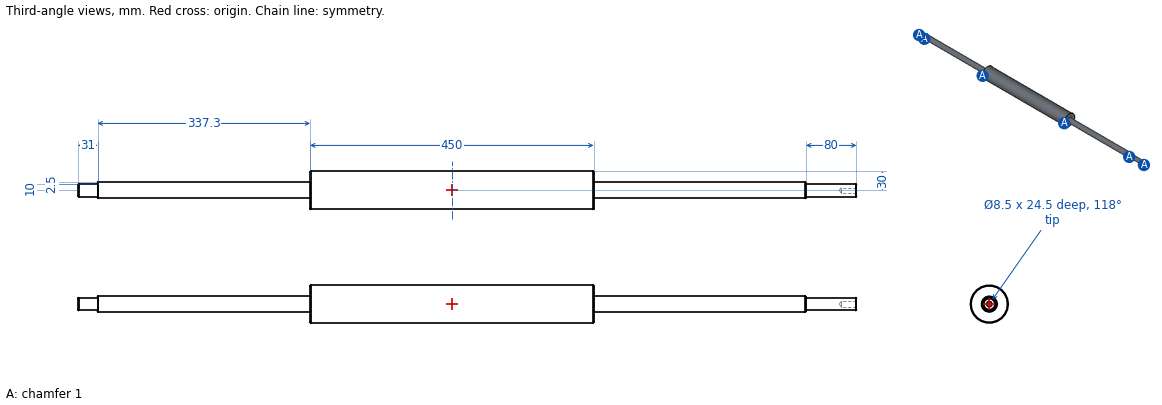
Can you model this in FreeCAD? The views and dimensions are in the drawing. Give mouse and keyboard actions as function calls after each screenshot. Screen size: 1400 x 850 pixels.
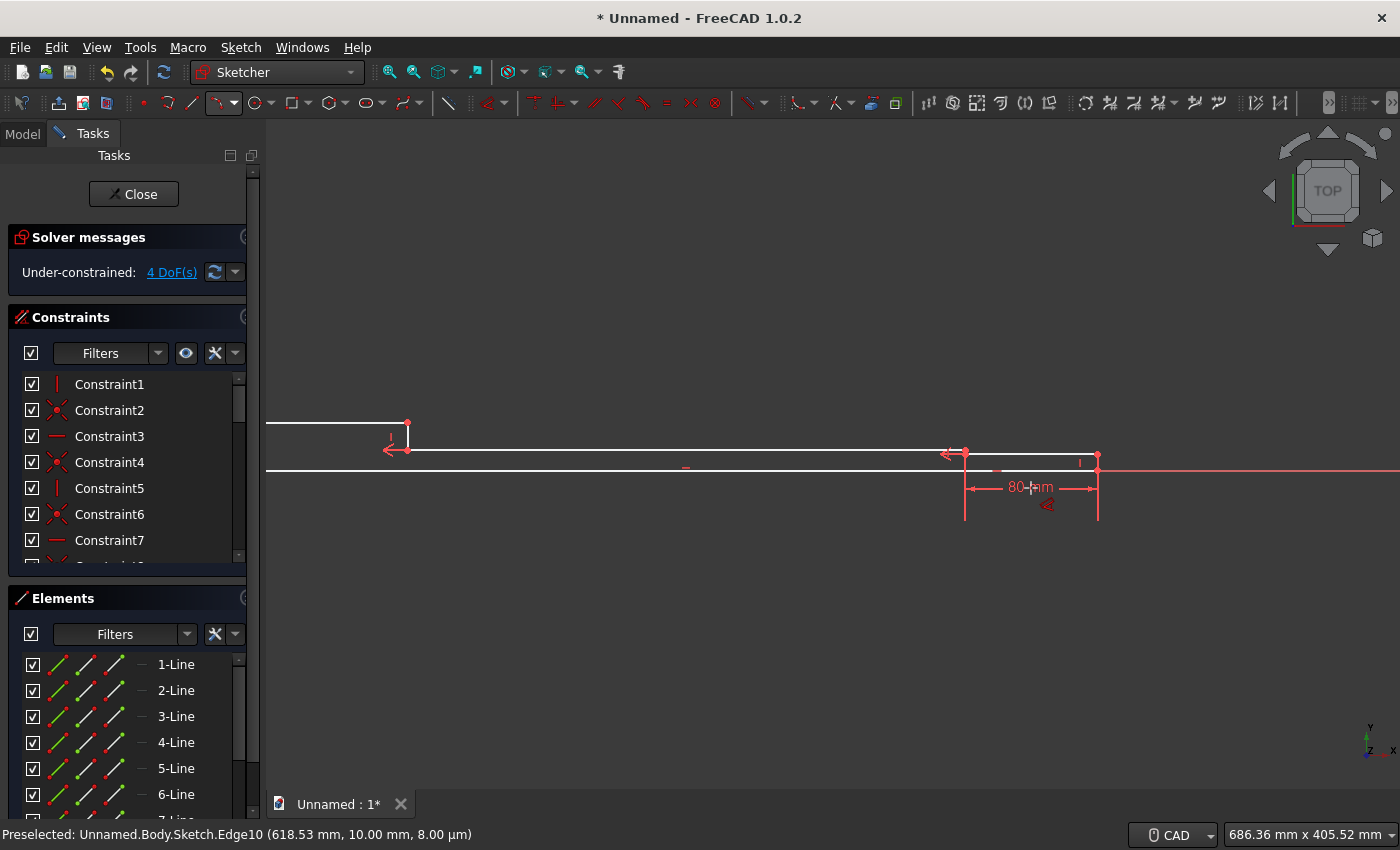
scroll(1061, 457, down, 6)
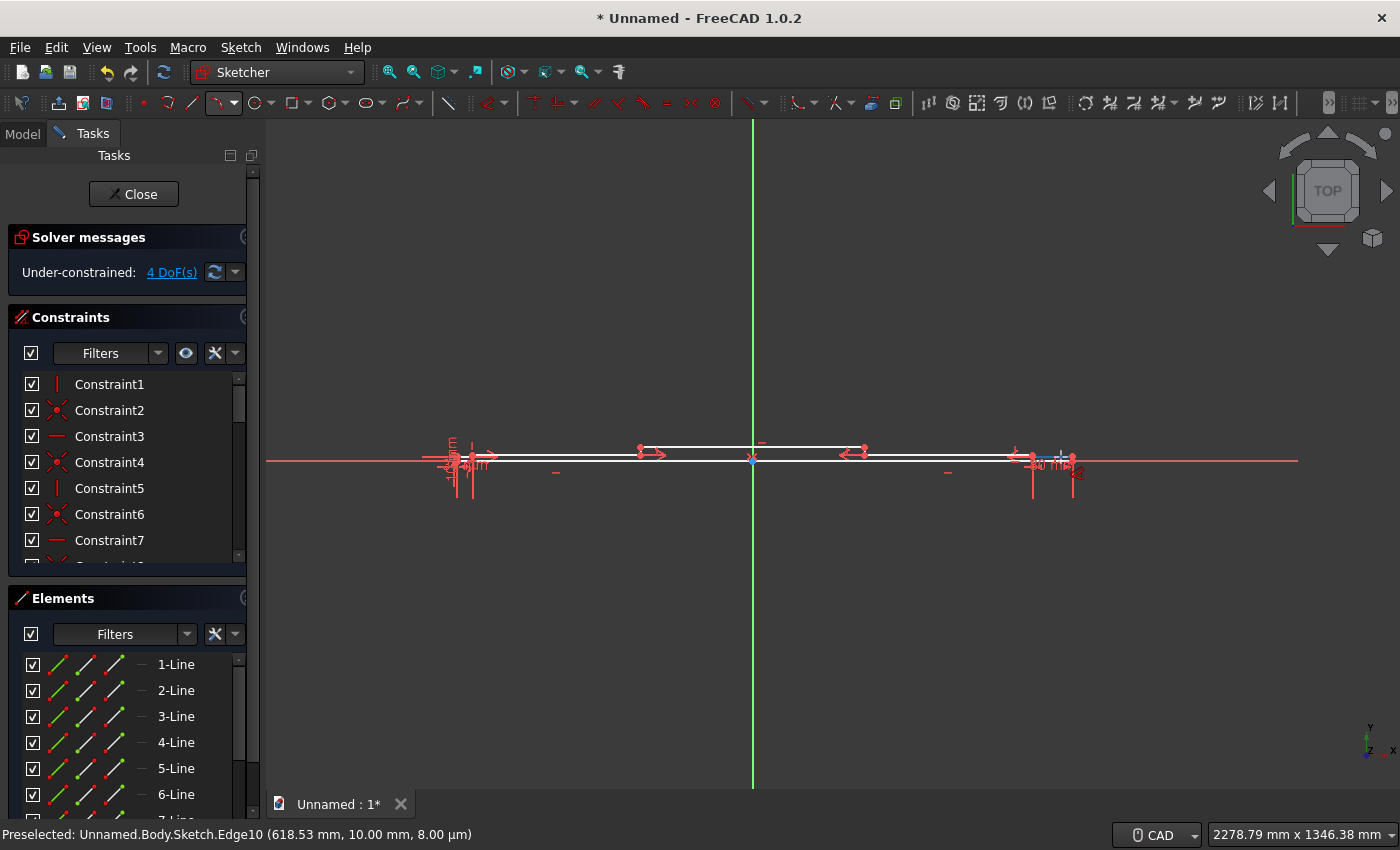
click(798, 447)
click(701, 413)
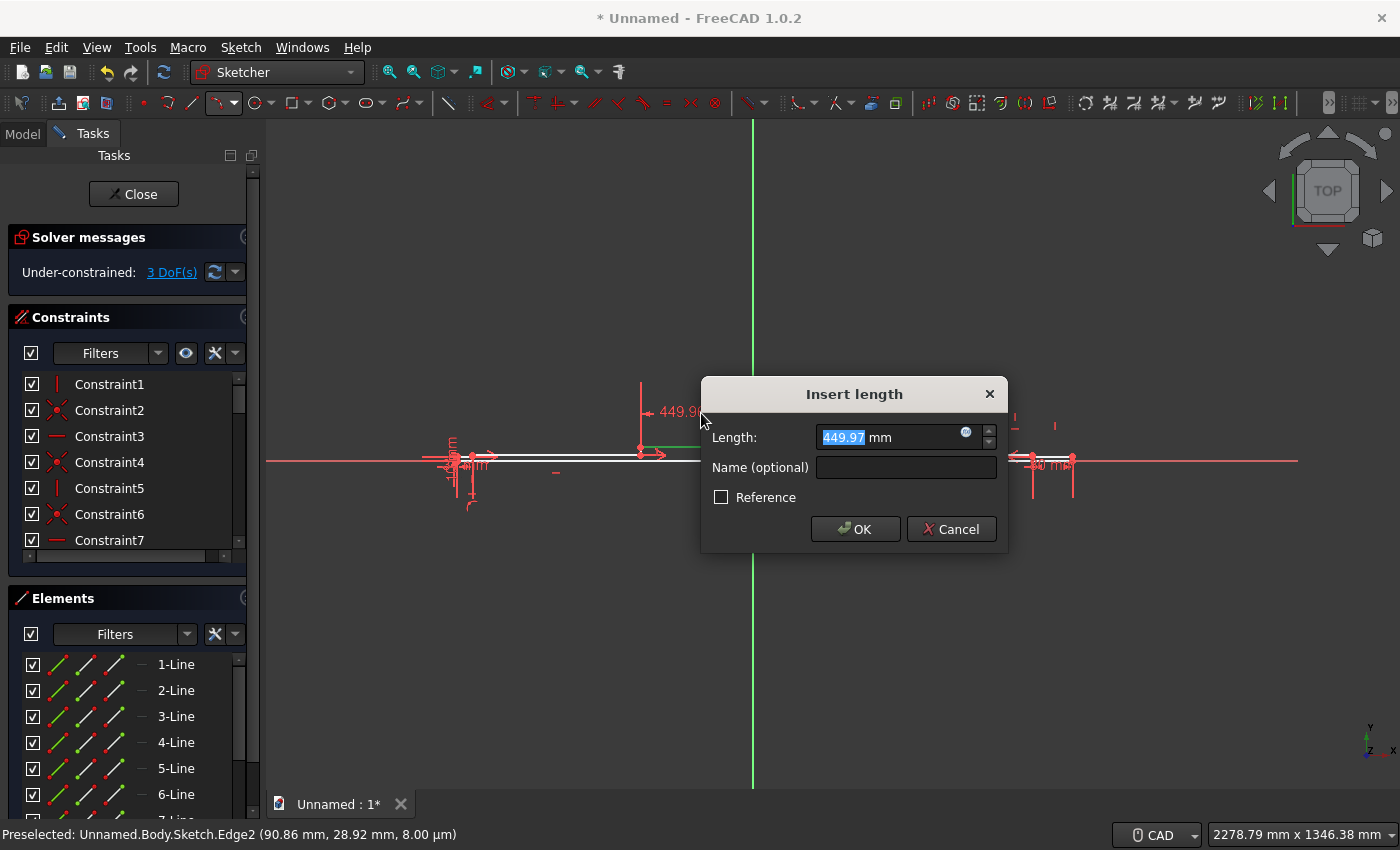
text(450)
key(Return)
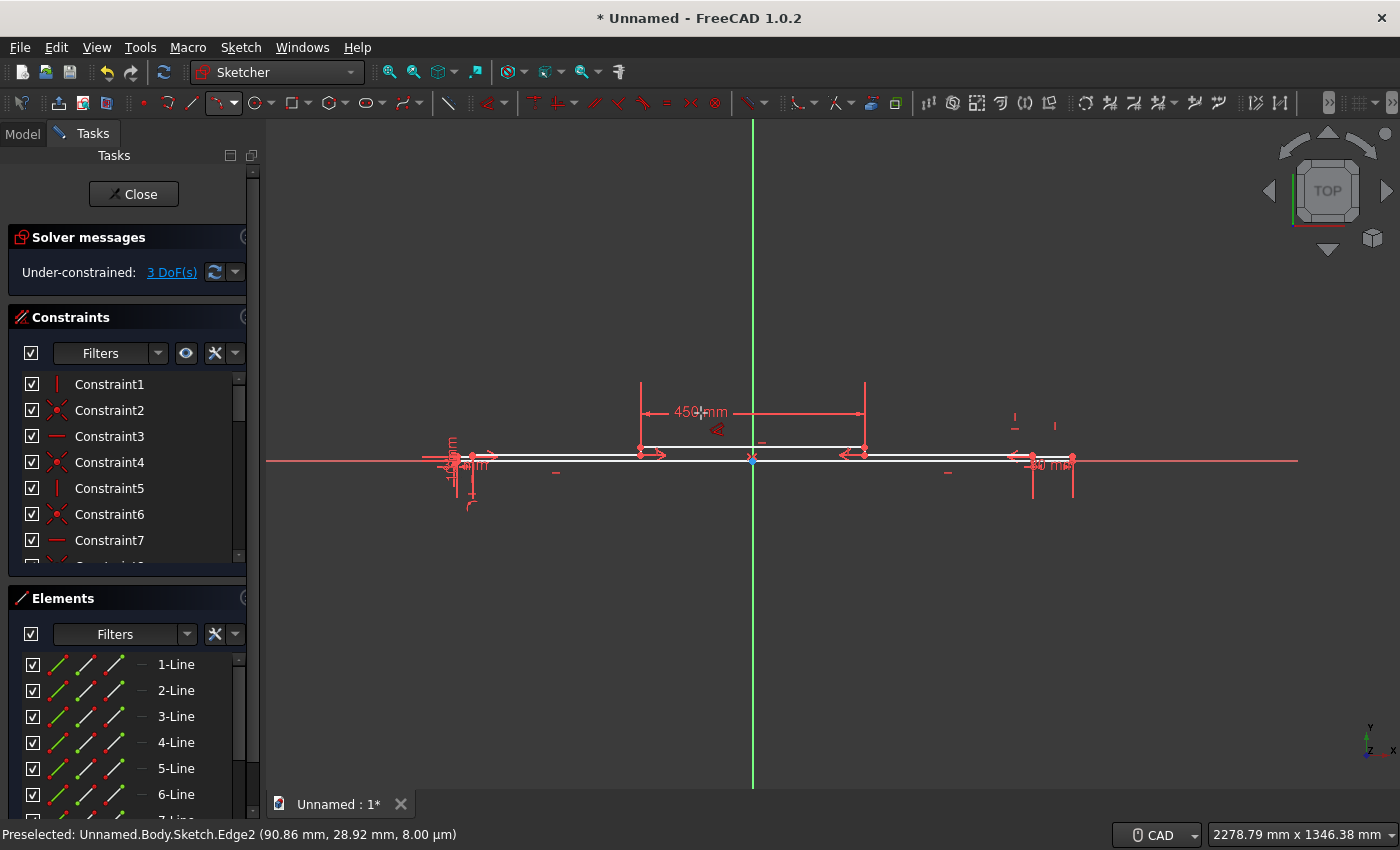
scroll(473, 456, up, 18)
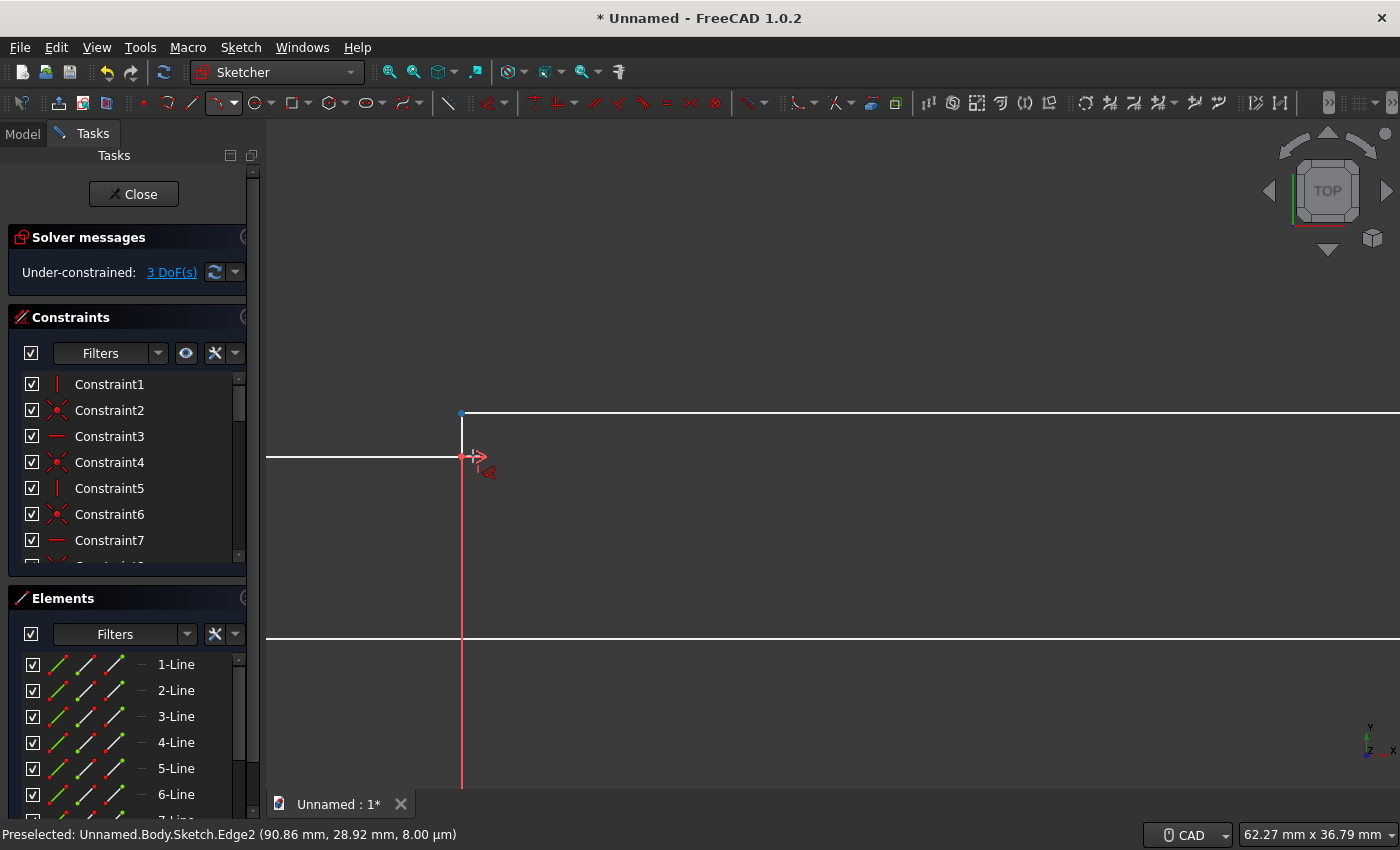
click(462, 435)
click(428, 435)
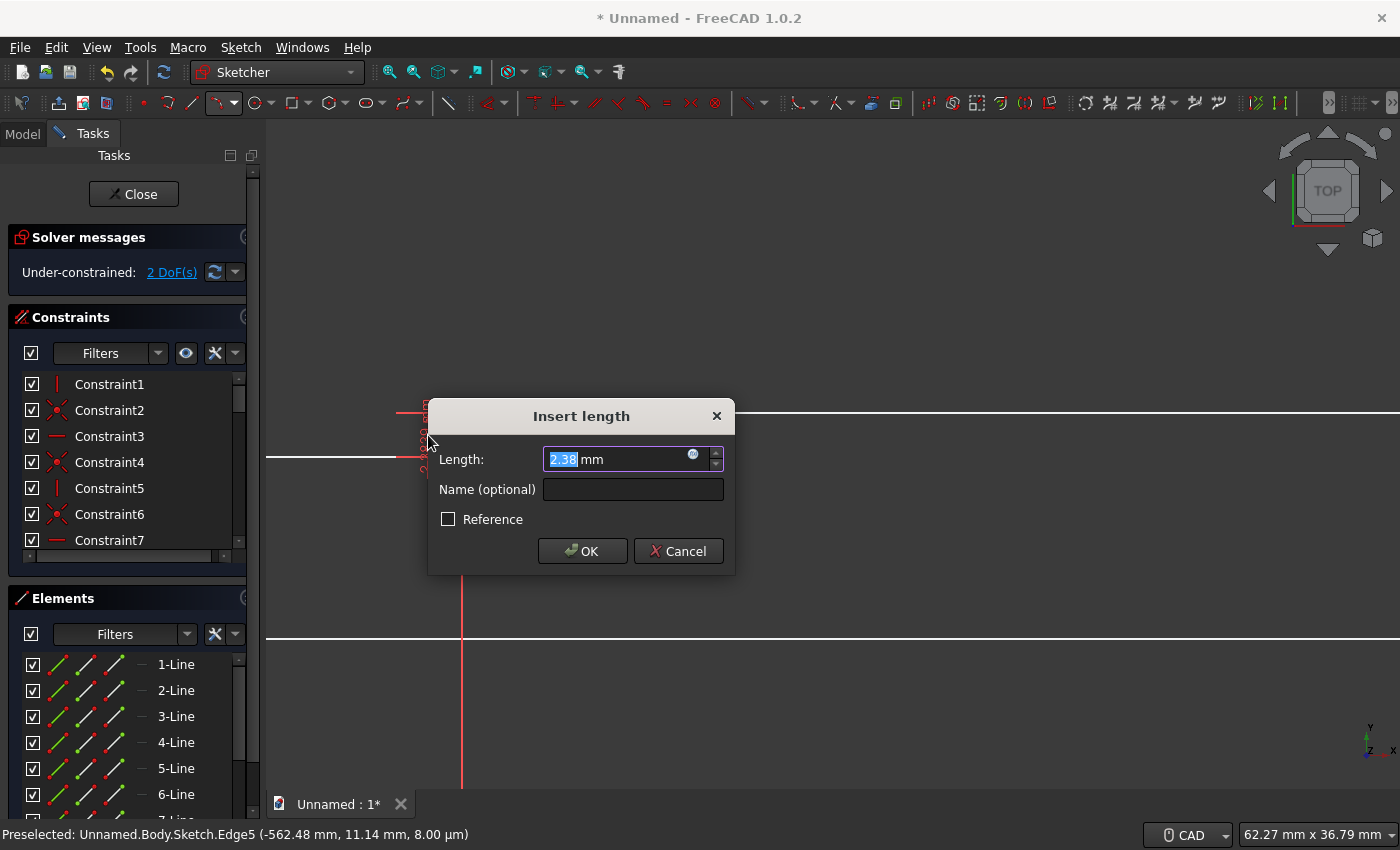
text(2.5)
key(Return)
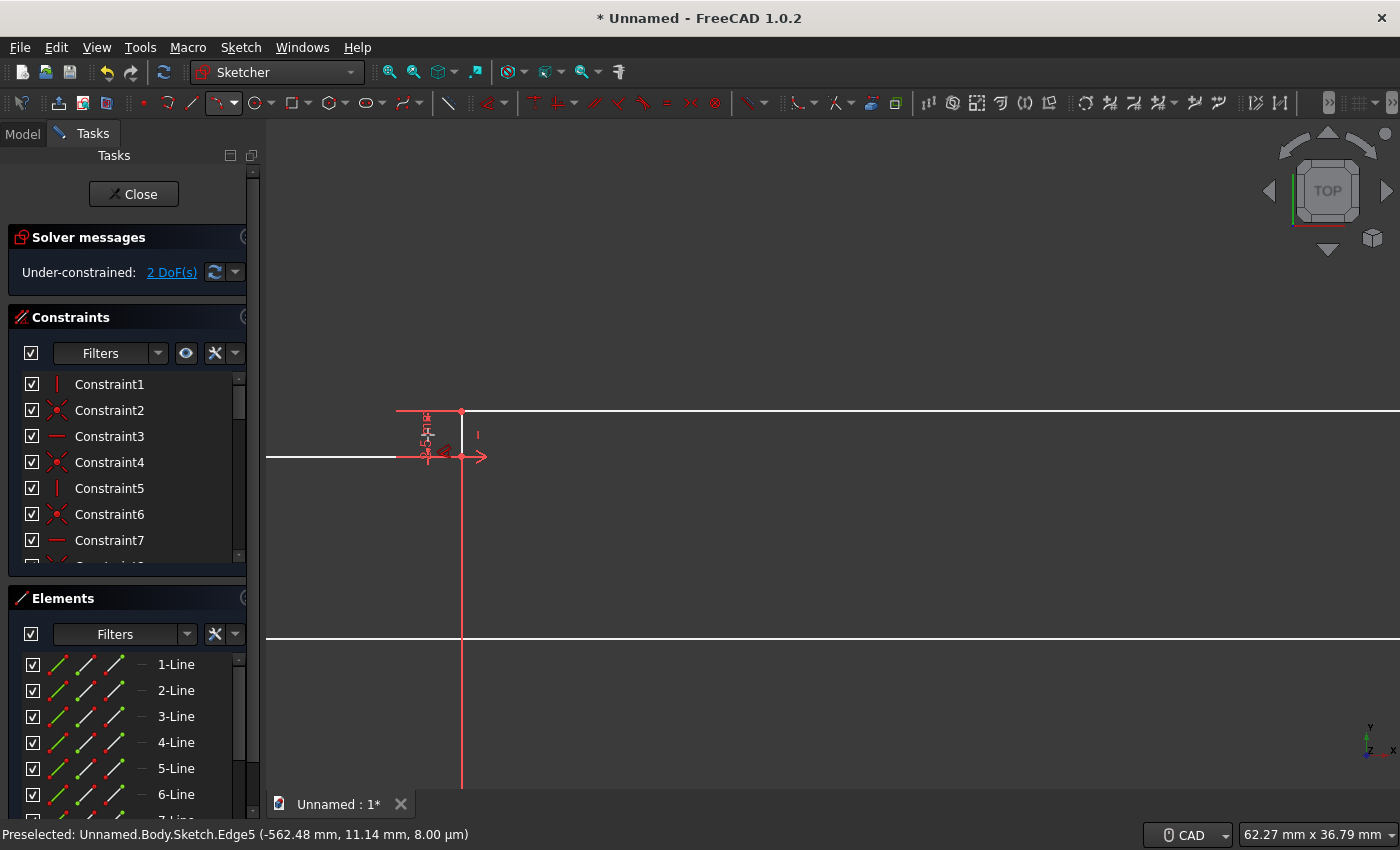
scroll(406, 457, down, 17)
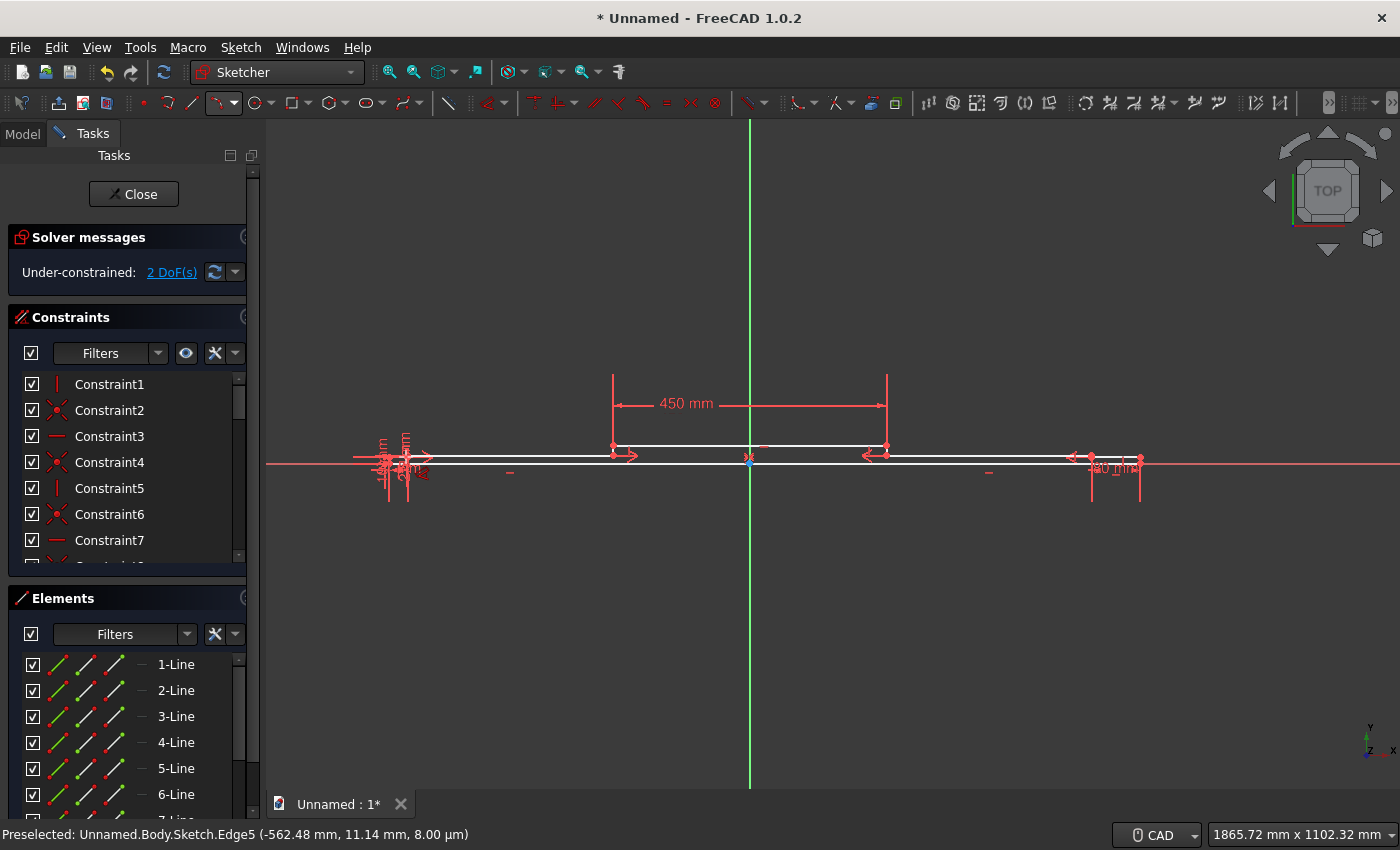
scroll(887, 446, up, 4)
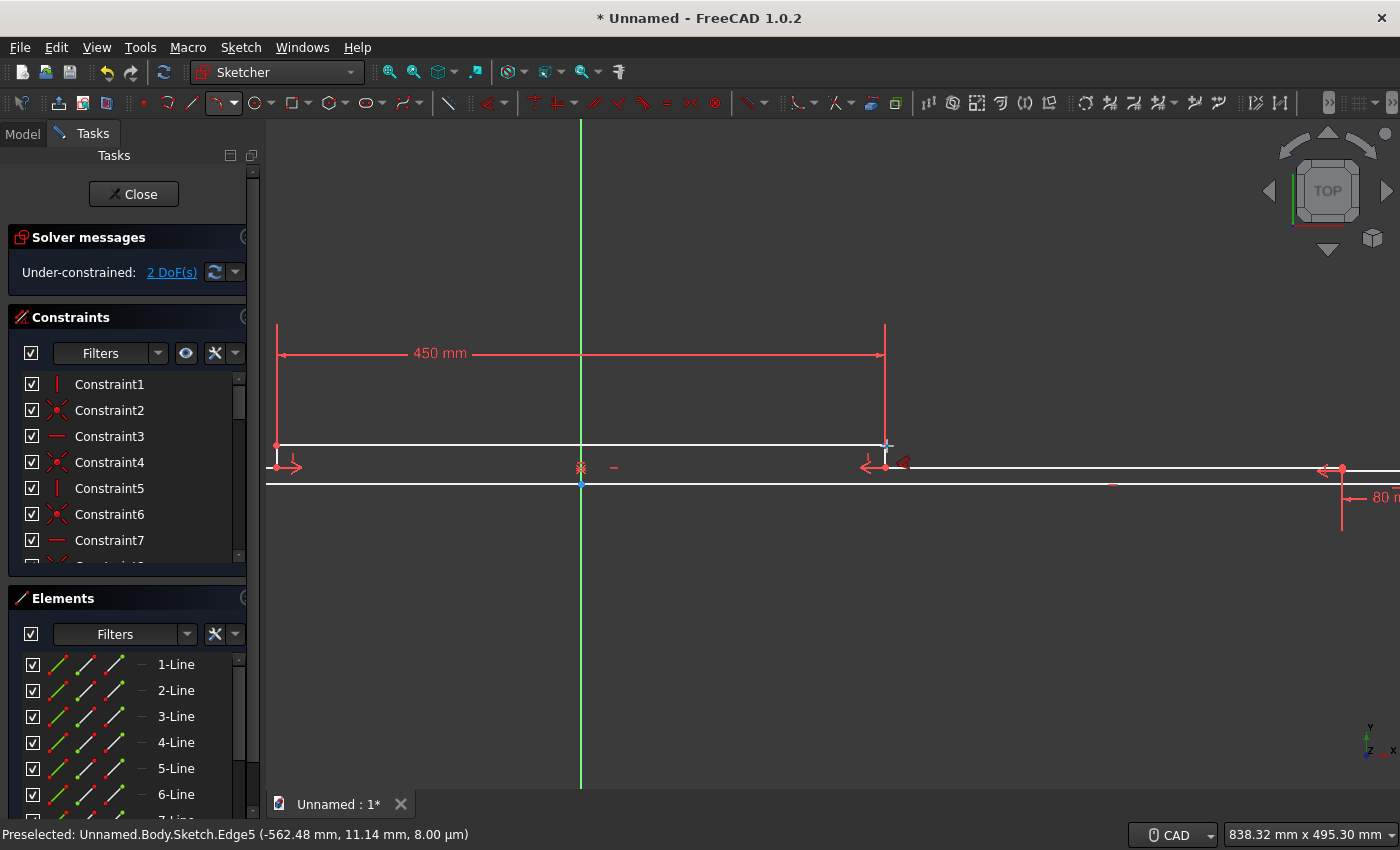
click(885, 445)
click(919, 451)